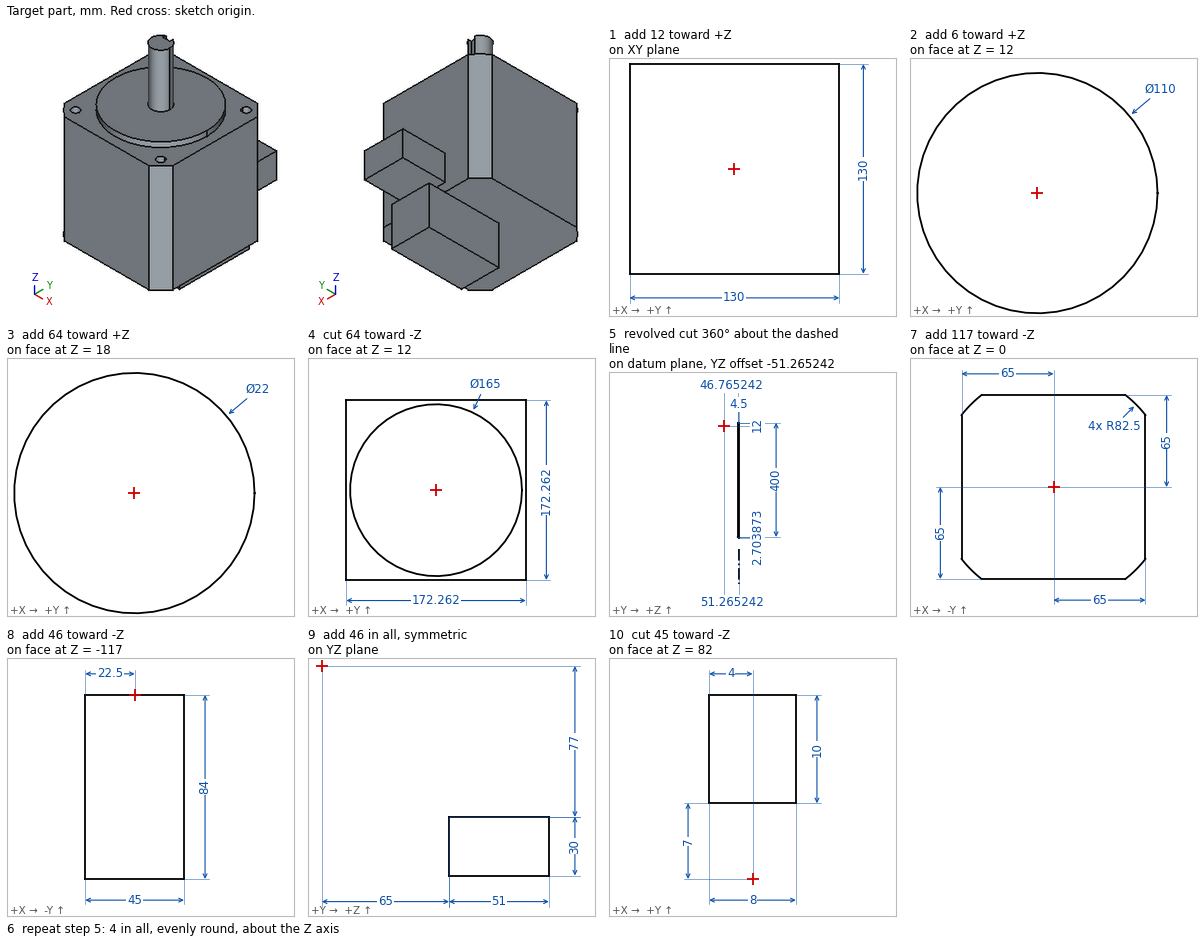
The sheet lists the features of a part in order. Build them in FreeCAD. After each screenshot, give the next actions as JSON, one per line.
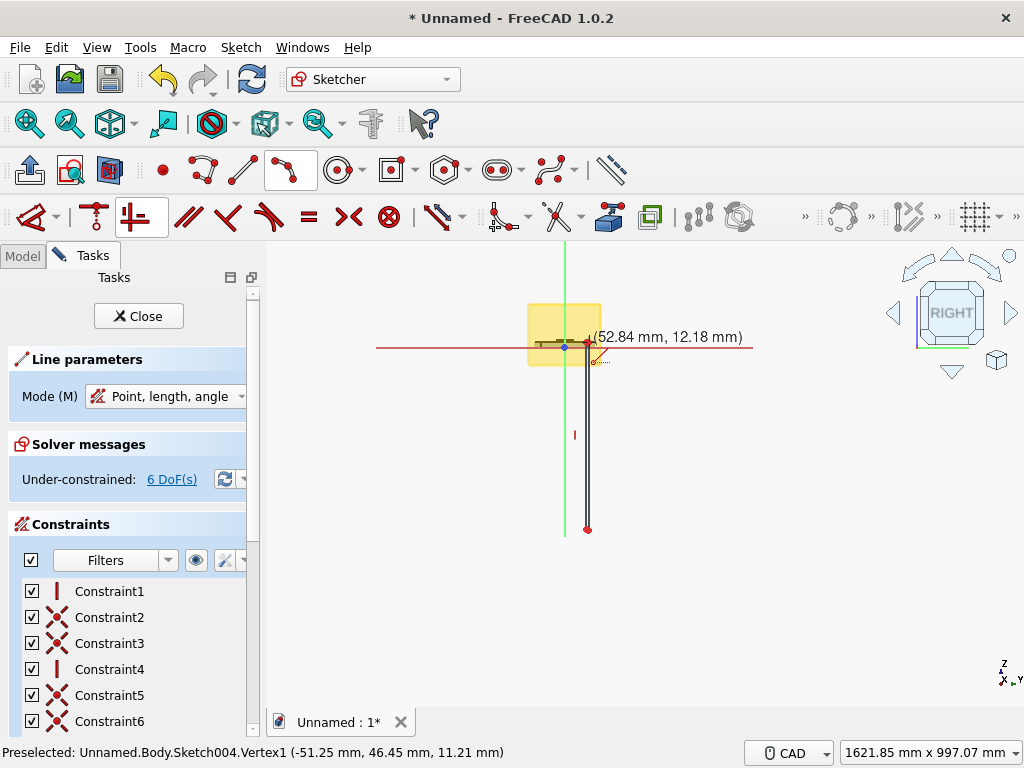
{"action": "left_click", "coordinate": [589, 549]}
{"action": "left_click", "coordinate": [589, 606]}
{"action": "key", "text": "Escape"}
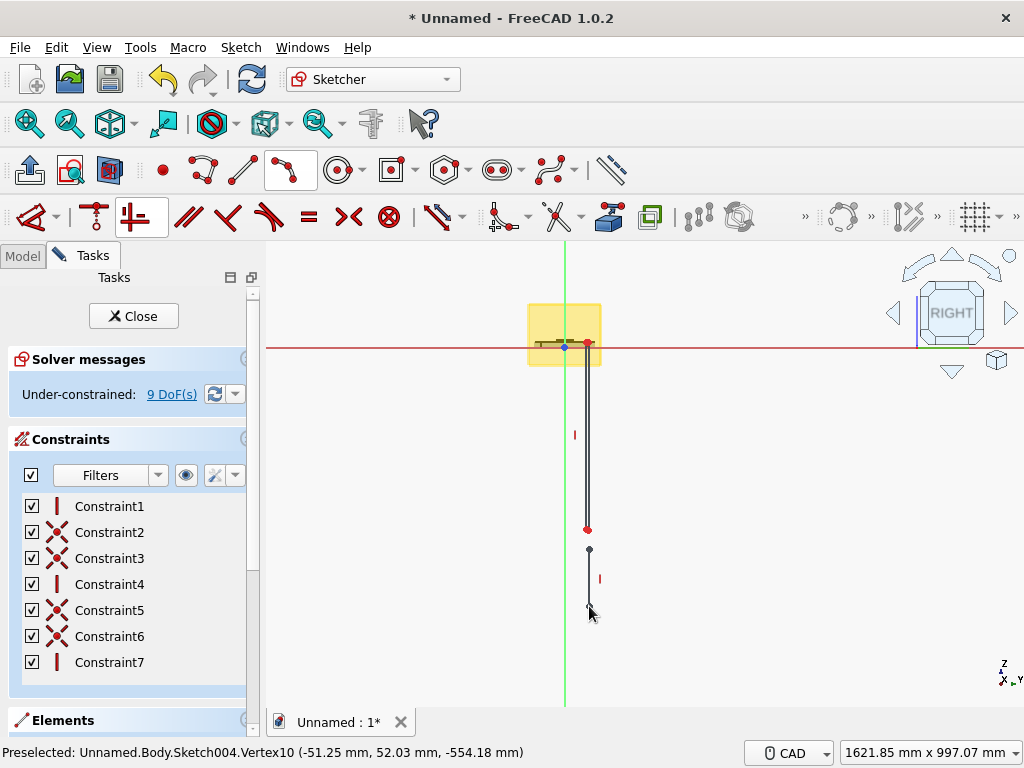
{"action": "left_click", "coordinate": [589, 567]}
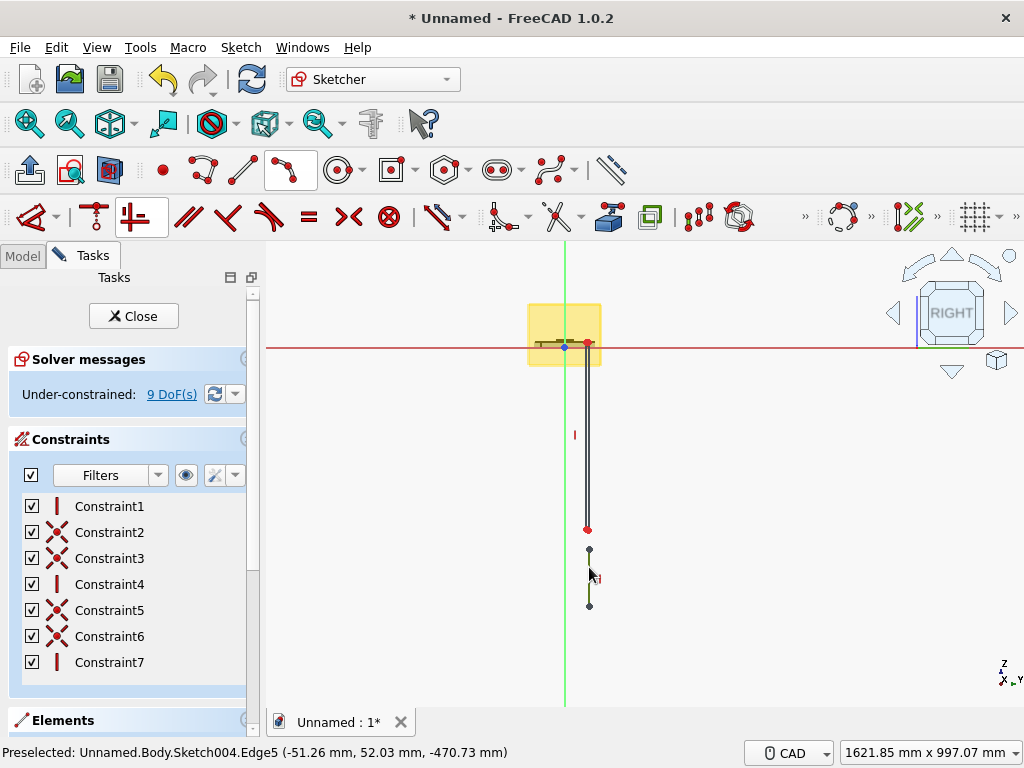
{"action": "left_click", "coordinate": [612, 170]}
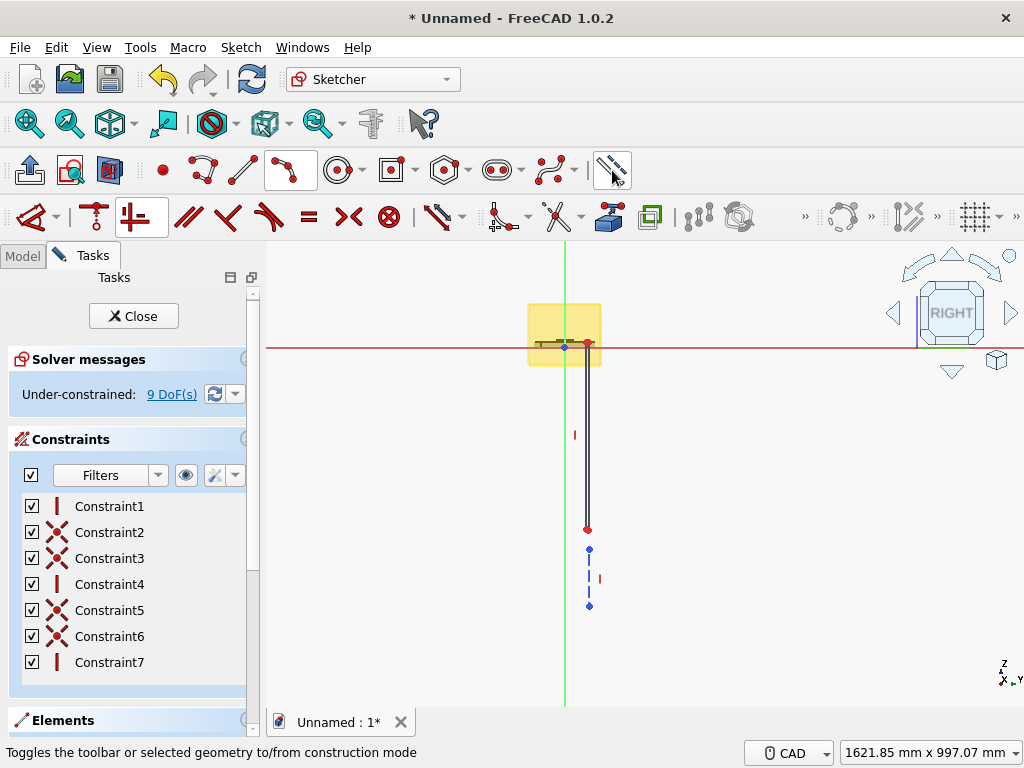
{"action": "scroll", "coordinate": [588, 343], "scroll_direction": "up", "scroll_amount": 13}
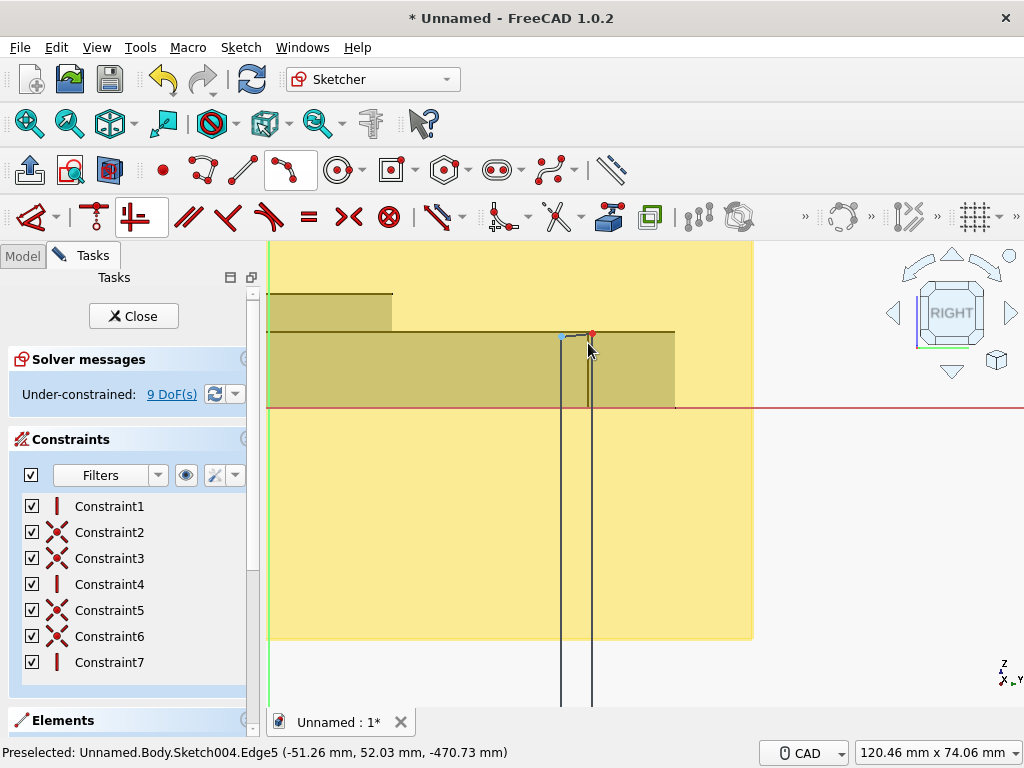
{"action": "left_click", "coordinate": [577, 335]}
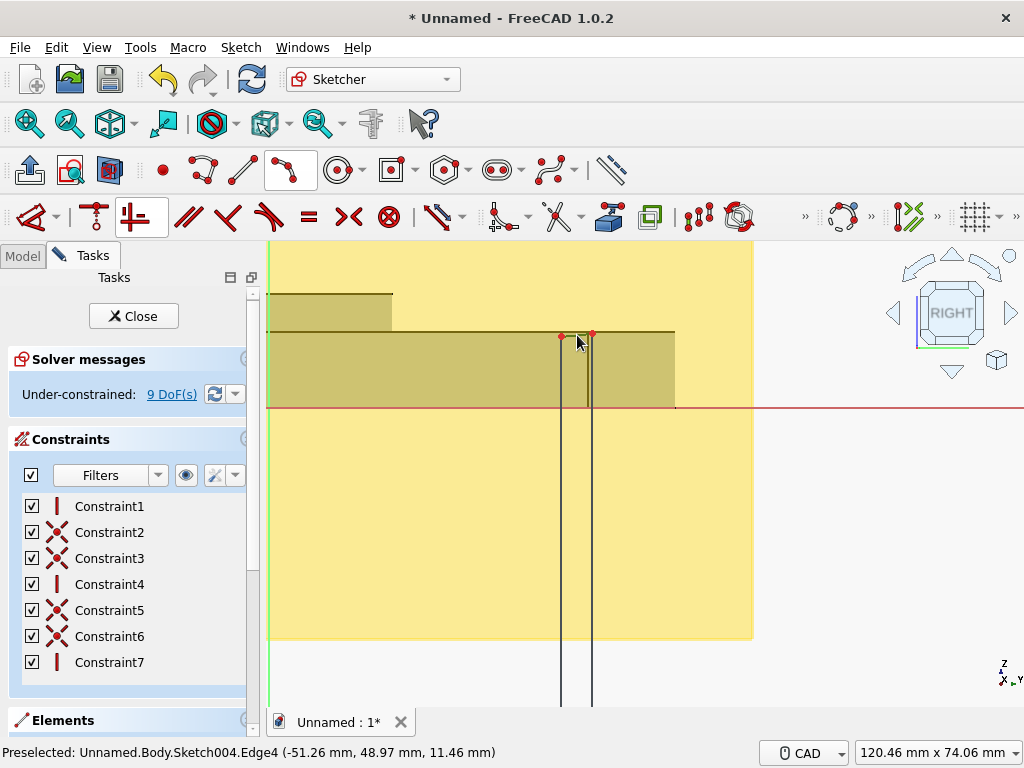
{"action": "left_click", "coordinate": [162, 218]}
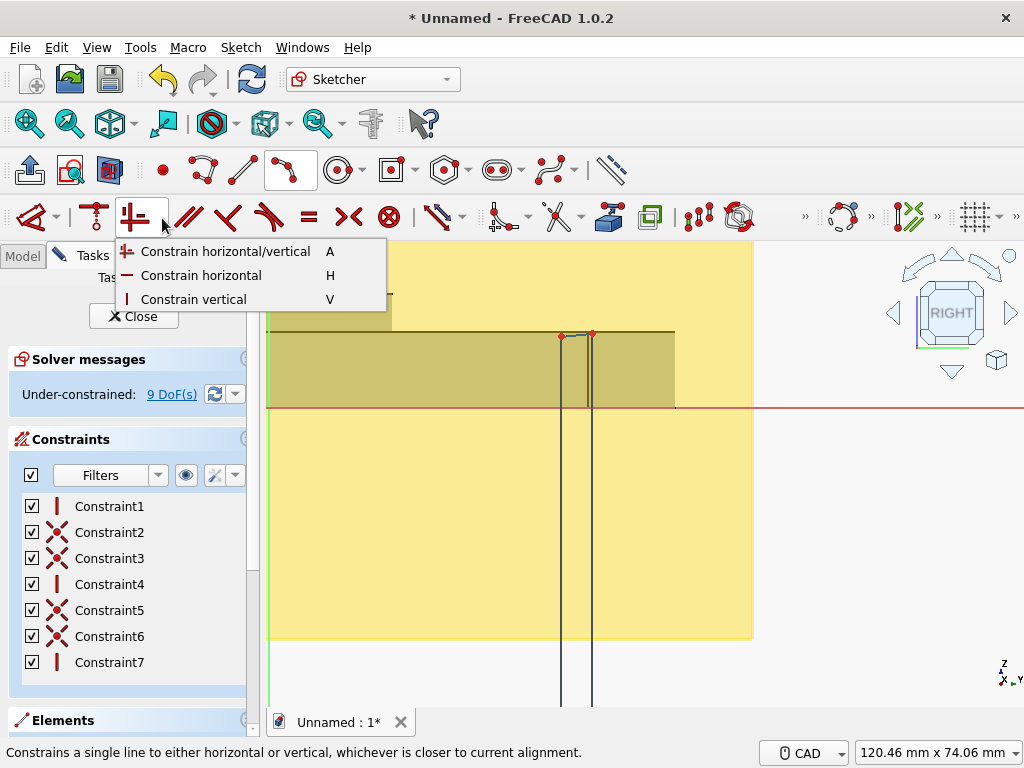
{"action": "left_click", "coordinate": [251, 275]}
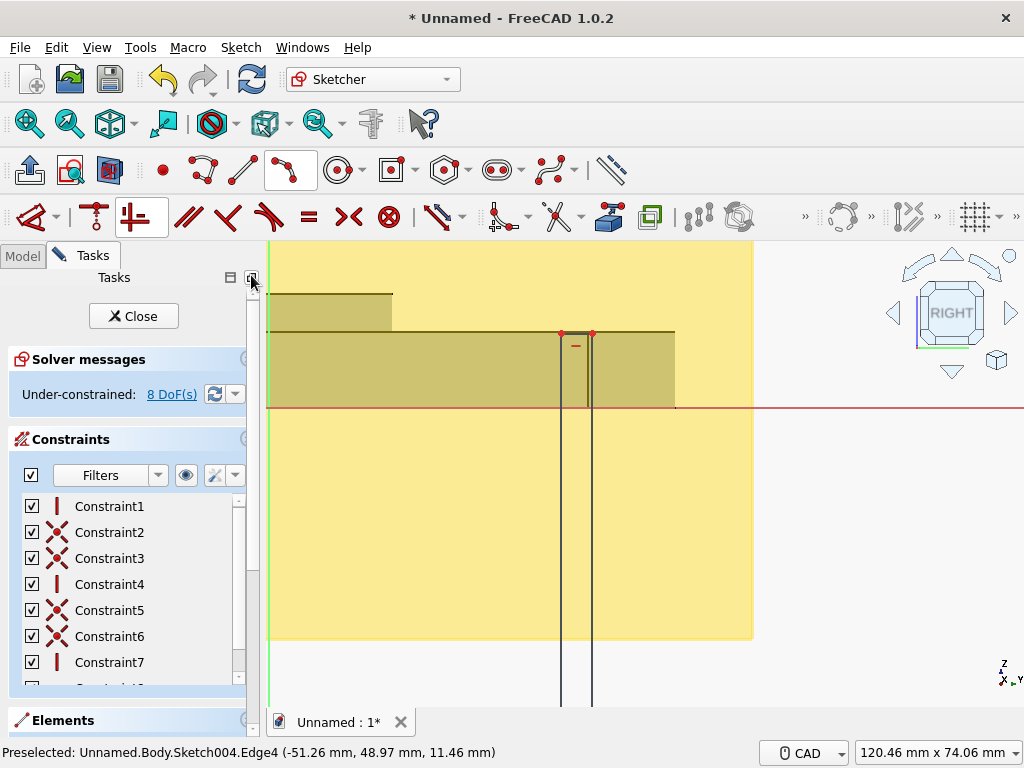
{"action": "left_click", "coordinate": [32, 218]}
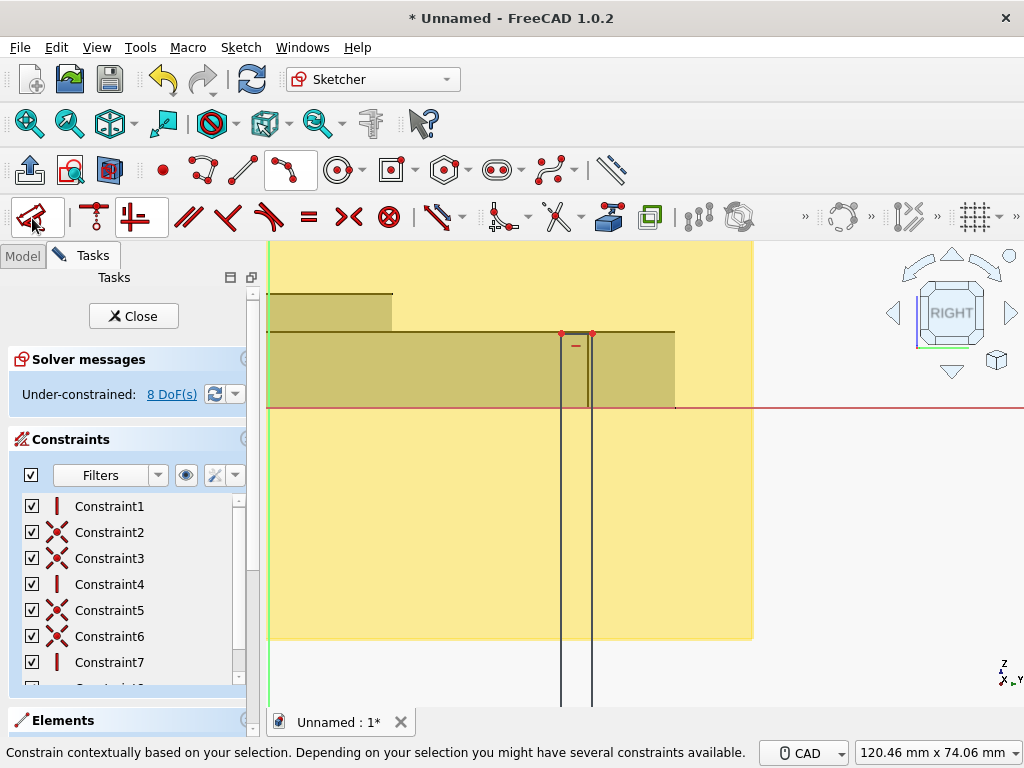
{"action": "scroll", "coordinate": [588, 343], "scroll_direction": "down", "scroll_amount": 13}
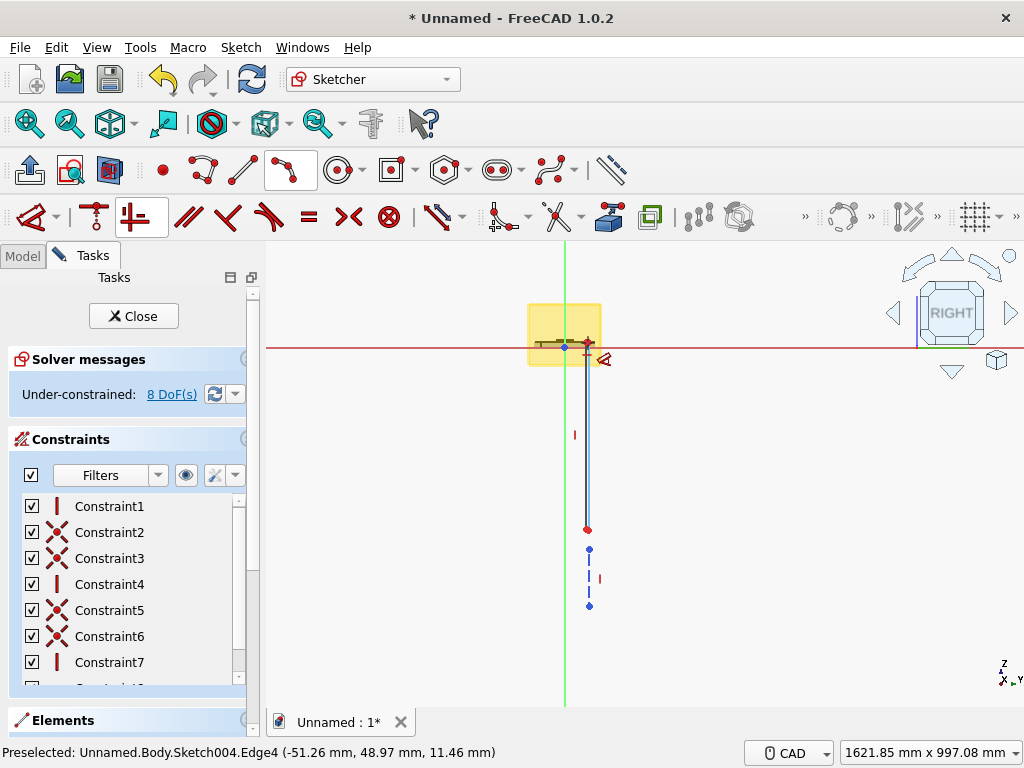
{"action": "scroll", "coordinate": [586, 399], "scroll_direction": "up", "scroll_amount": 9}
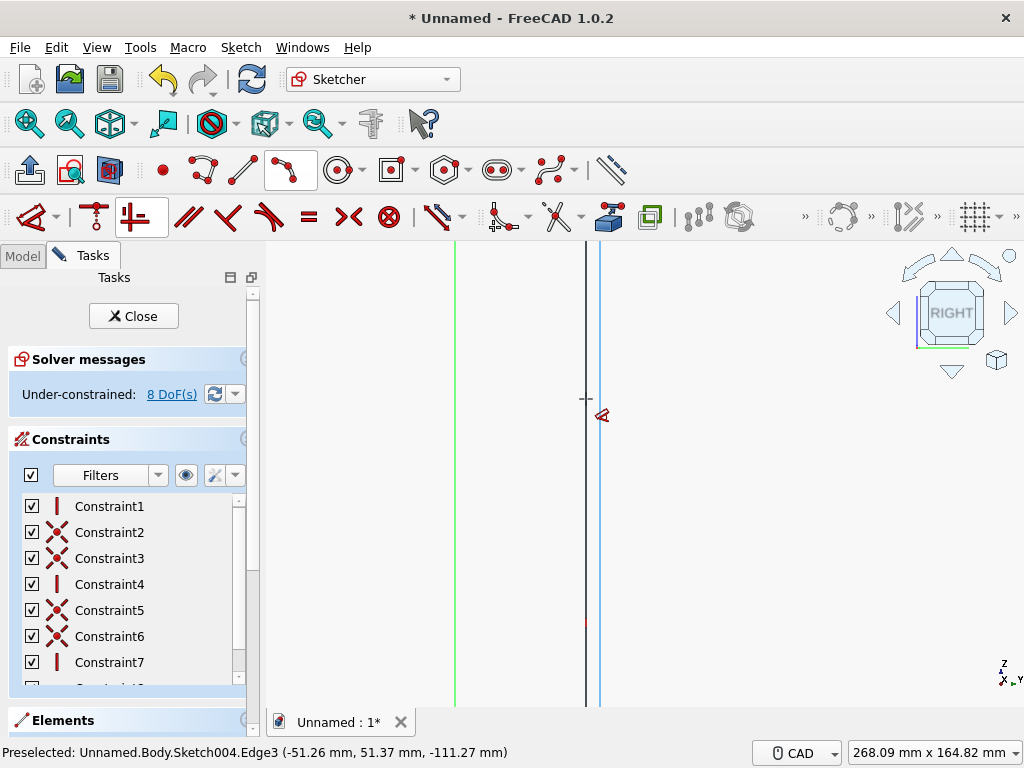
{"action": "left_click", "coordinate": [586, 396]}
{"action": "left_click", "coordinate": [620, 474]}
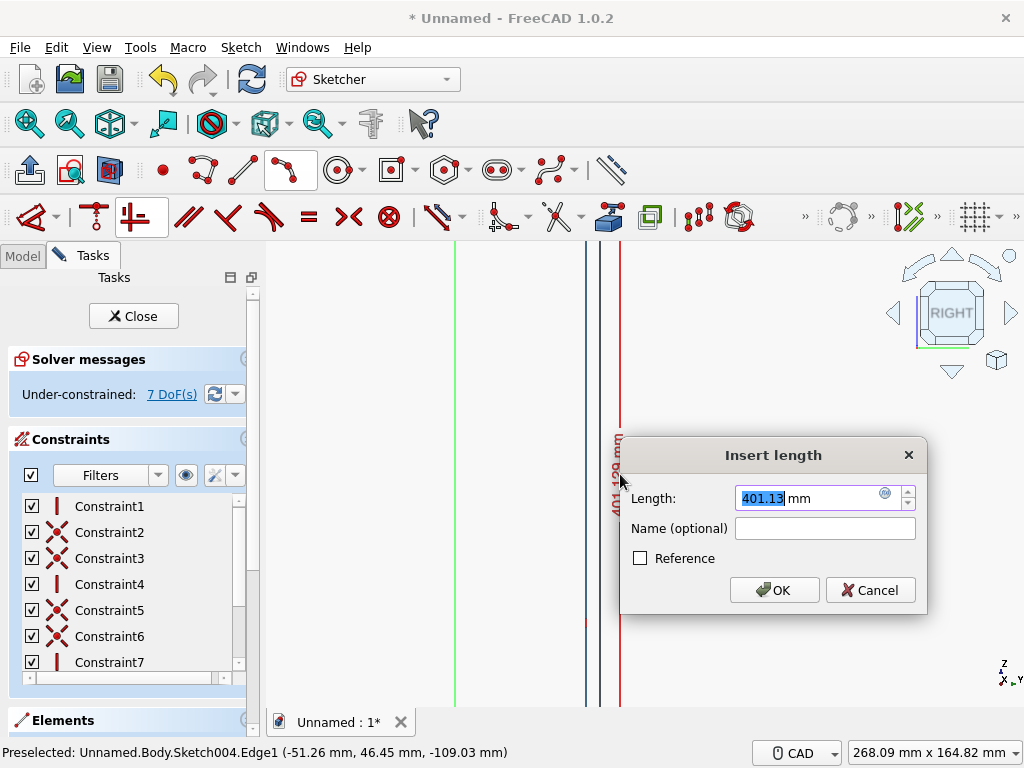
{"action": "type", "text": "400"}
{"action": "key", "text": "Return"}